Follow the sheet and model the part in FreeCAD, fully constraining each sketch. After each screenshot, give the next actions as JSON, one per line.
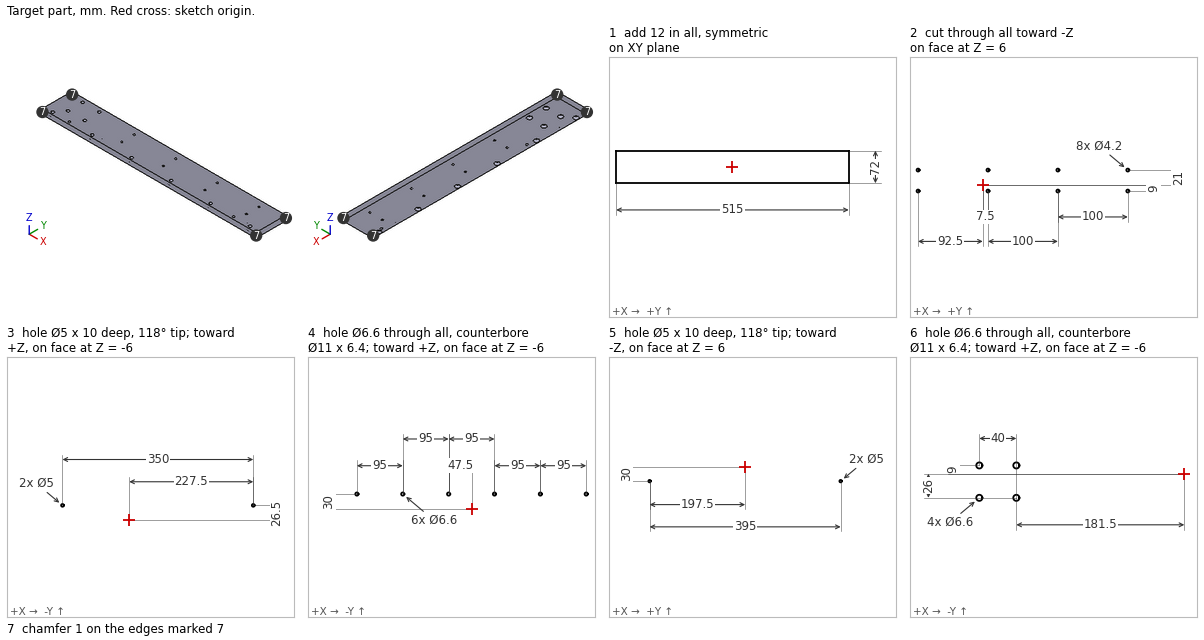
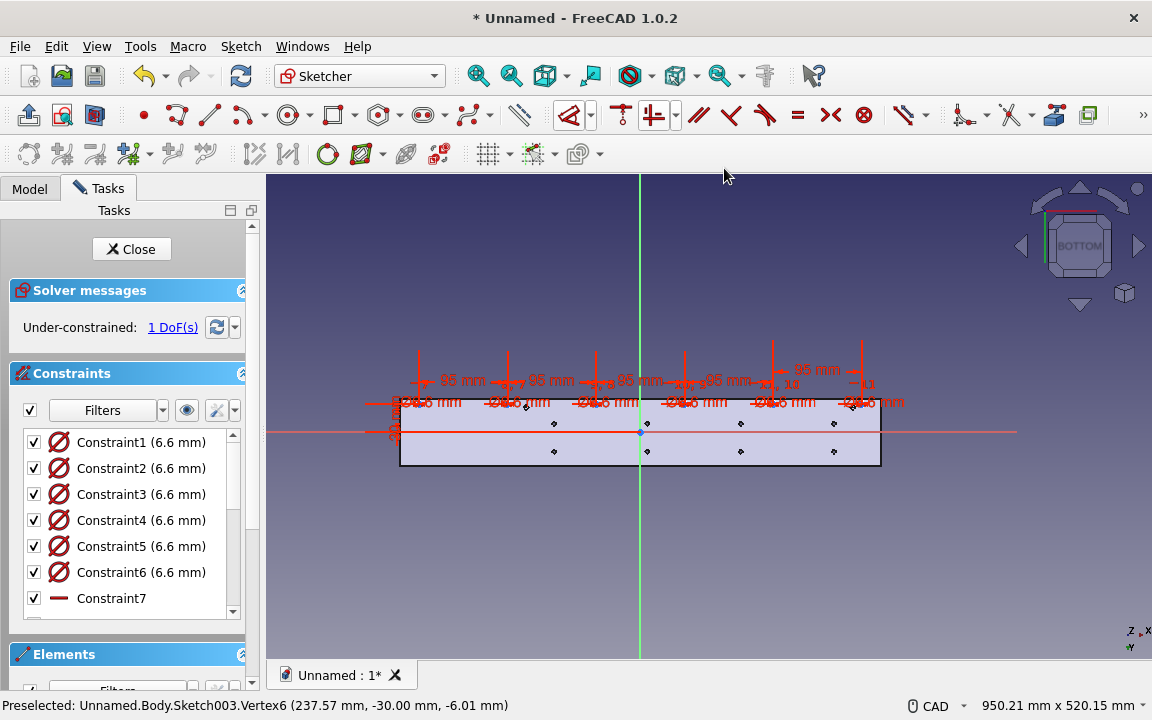
{"action": "left_click", "coordinate": [596, 404]}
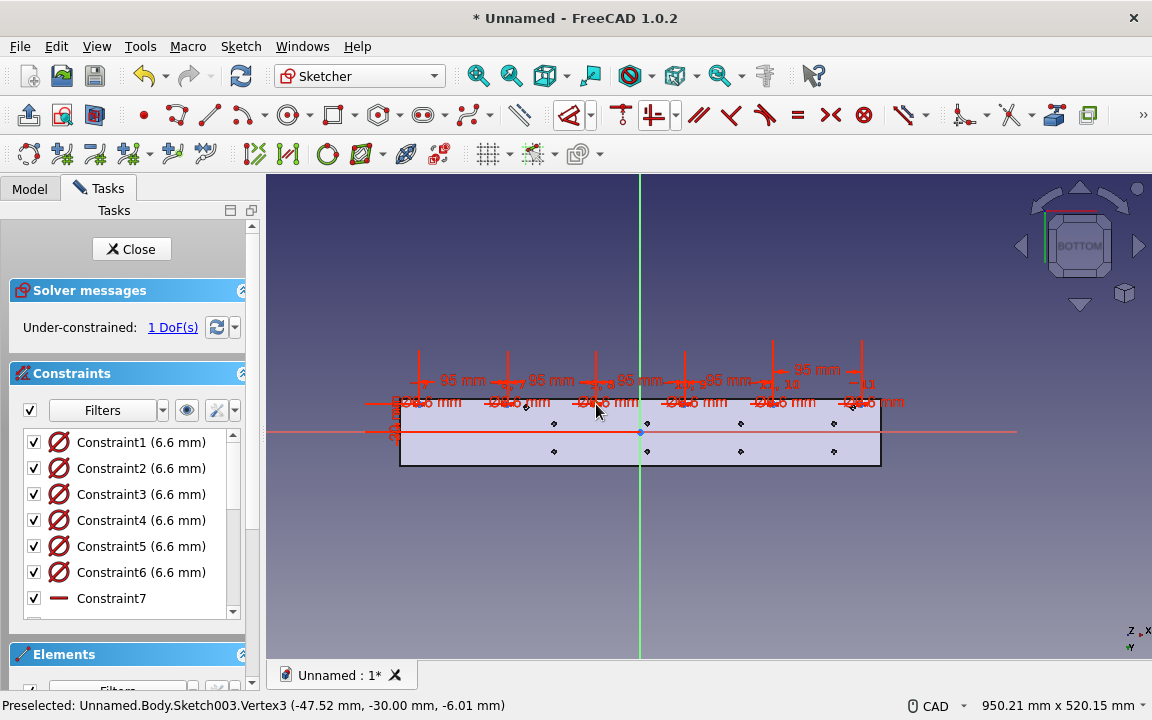
{"action": "left_click", "coordinate": [590, 116]}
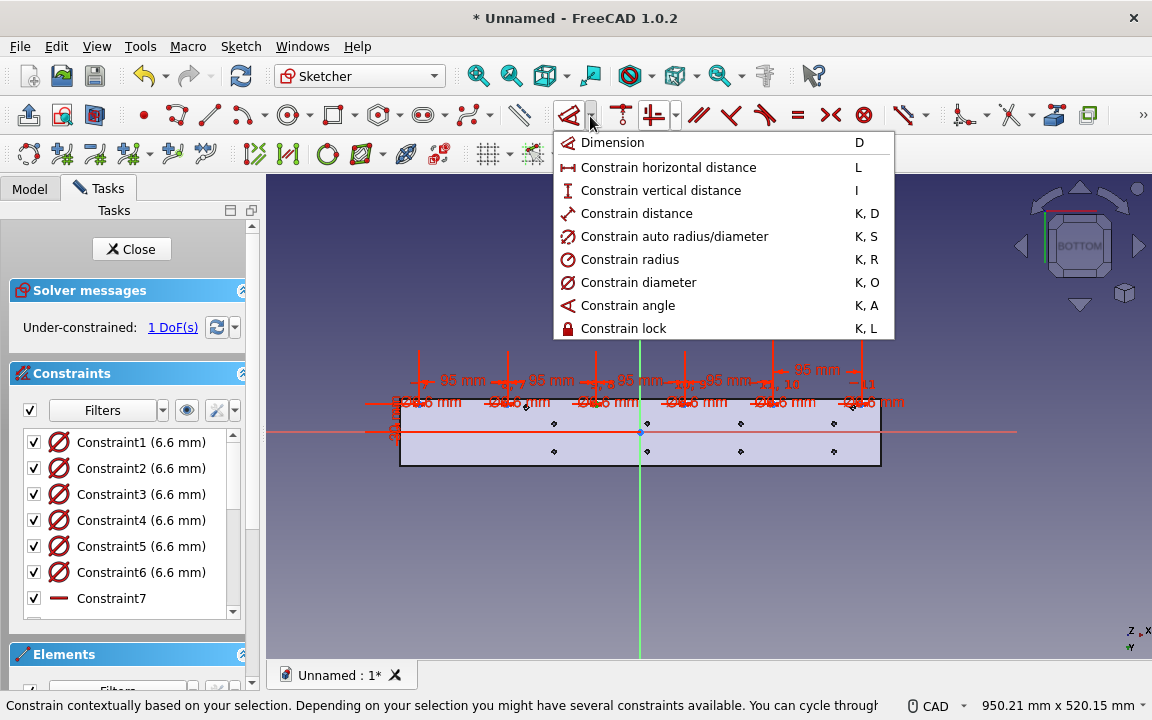
{"action": "left_click", "coordinate": [724, 168]}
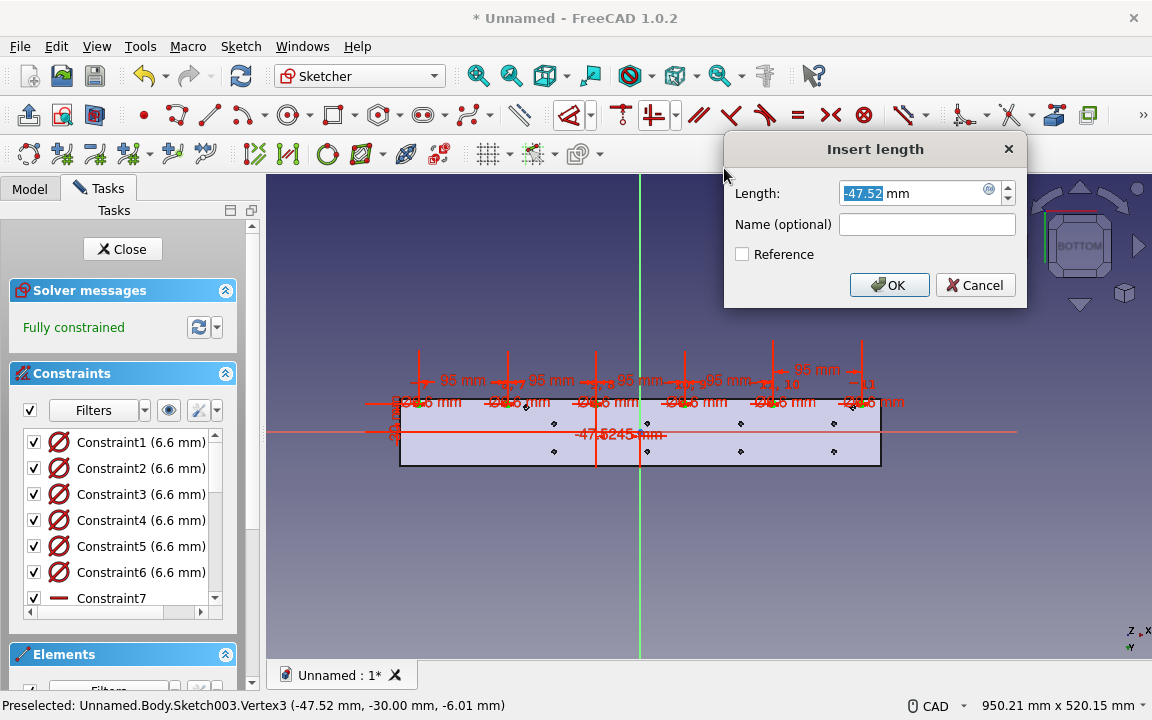
{"action": "type", "text": "-47.5"}
{"action": "key", "text": "Return"}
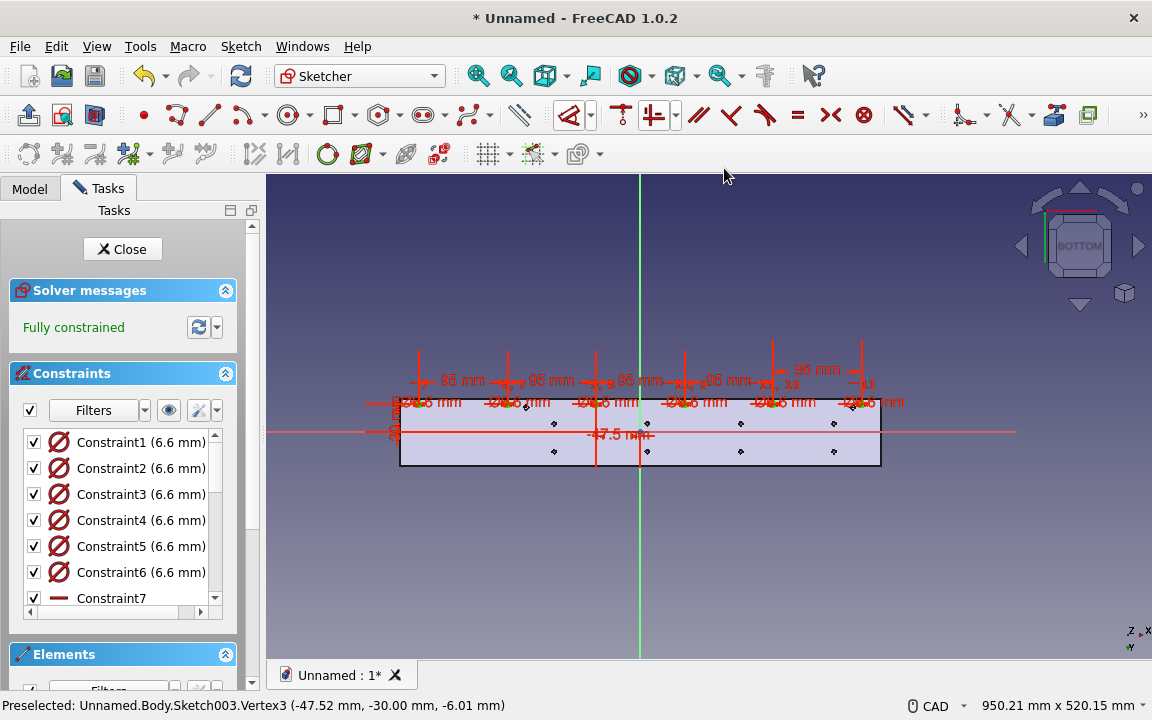
{"action": "left_click", "coordinate": [123, 249]}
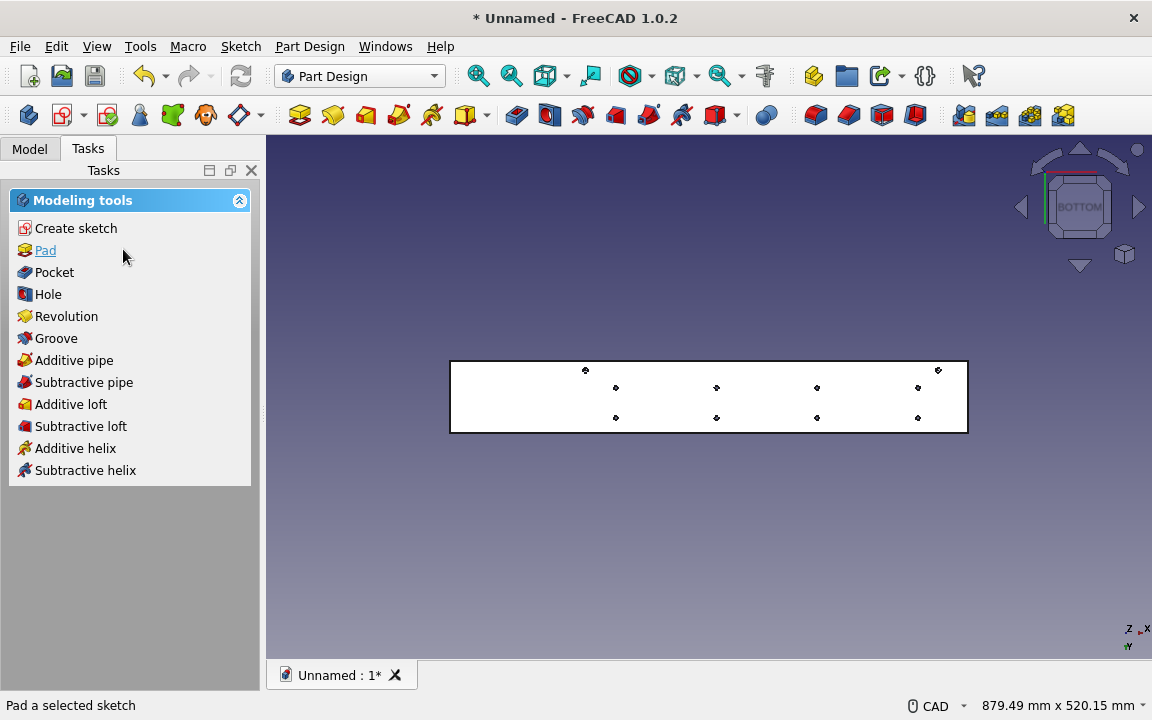
{"action": "left_click", "coordinate": [550, 116]}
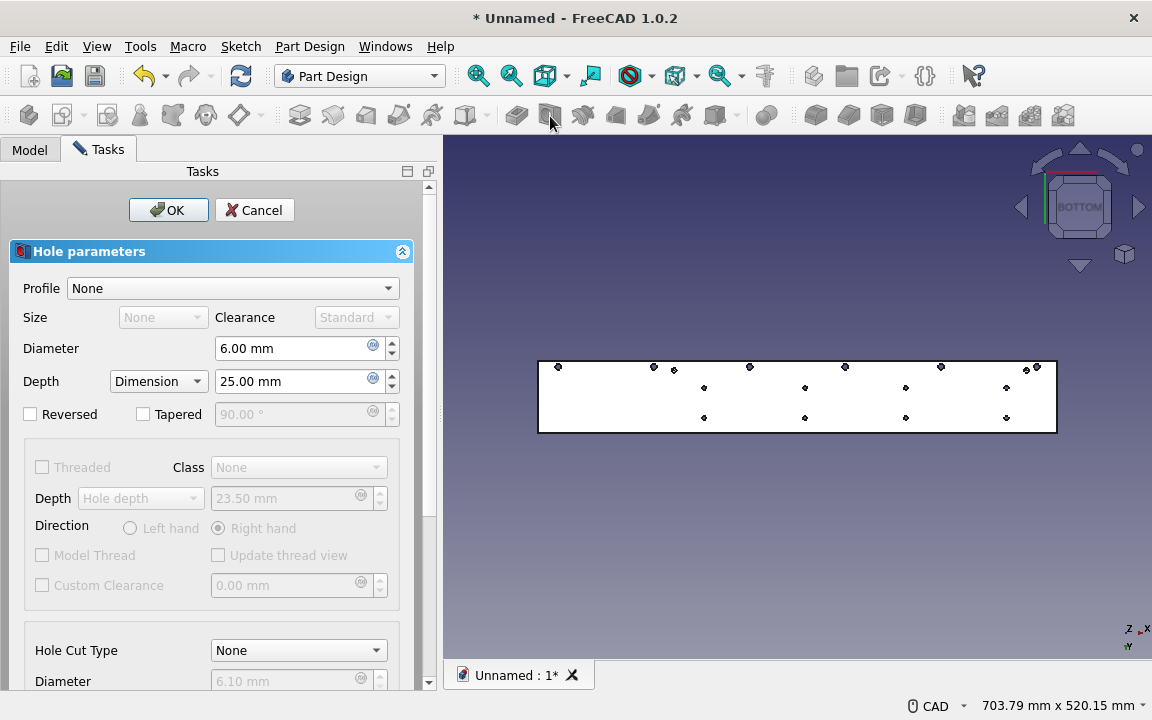
{"action": "triple_click", "coordinate": [300, 348]}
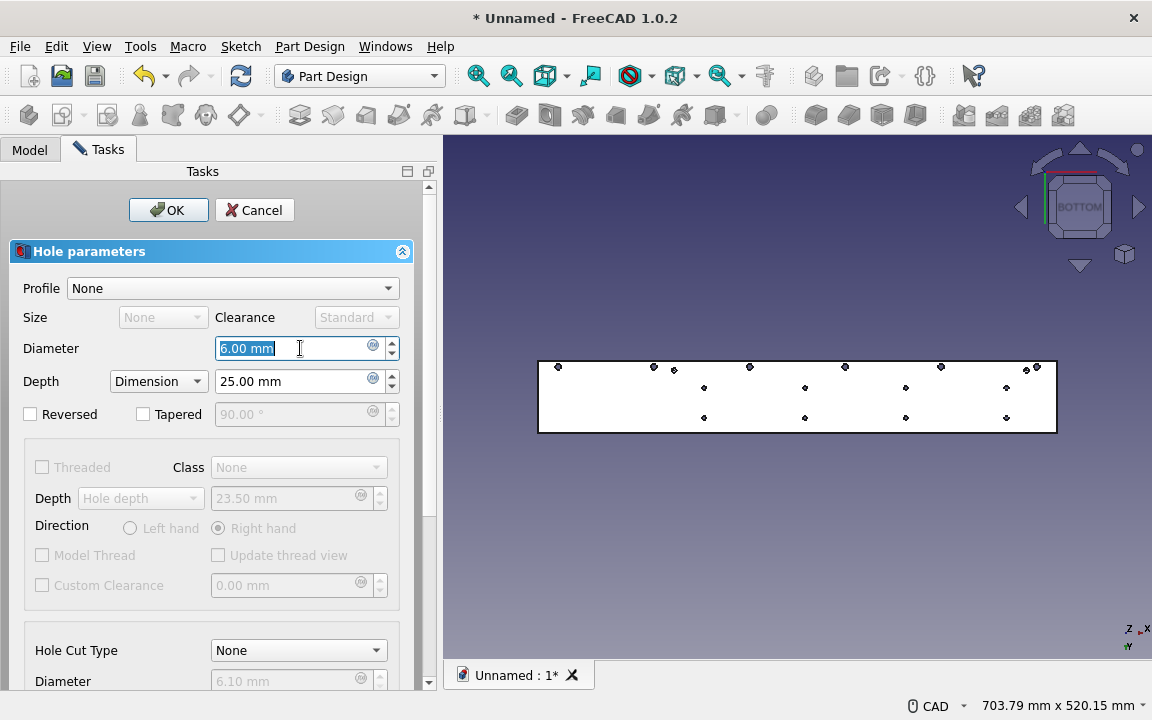
{"action": "type", "text": "6.6"}
{"action": "key", "text": "Tab"}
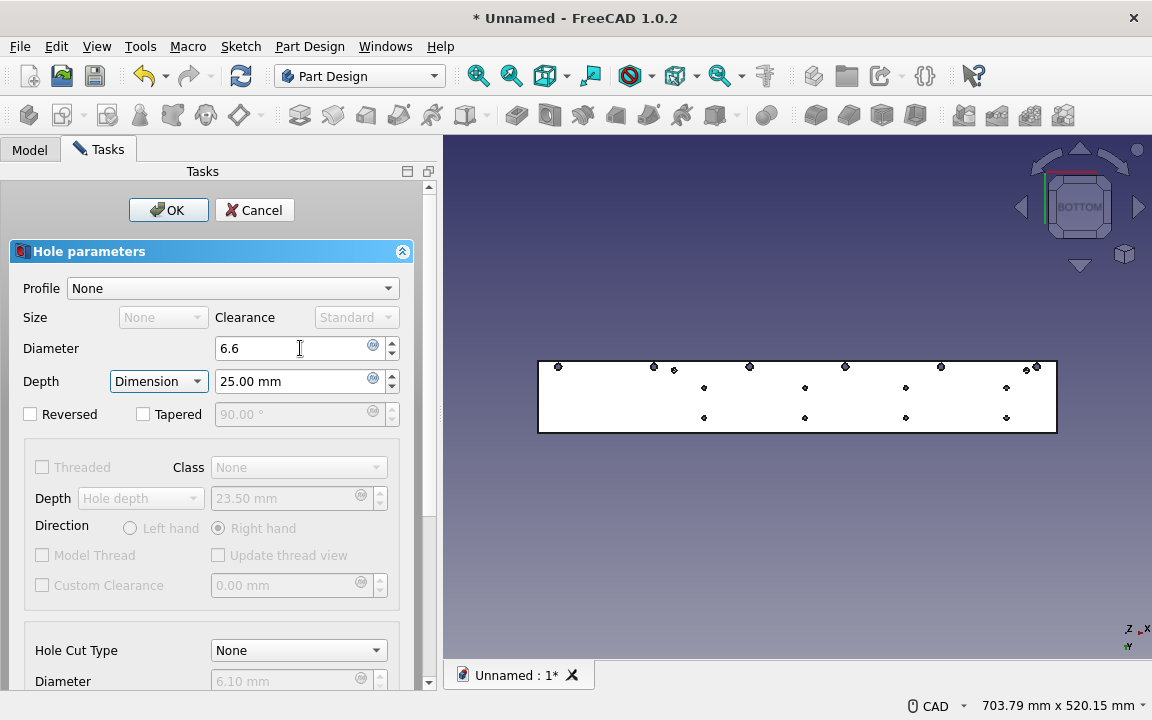
{"action": "left_click", "coordinate": [160, 382]}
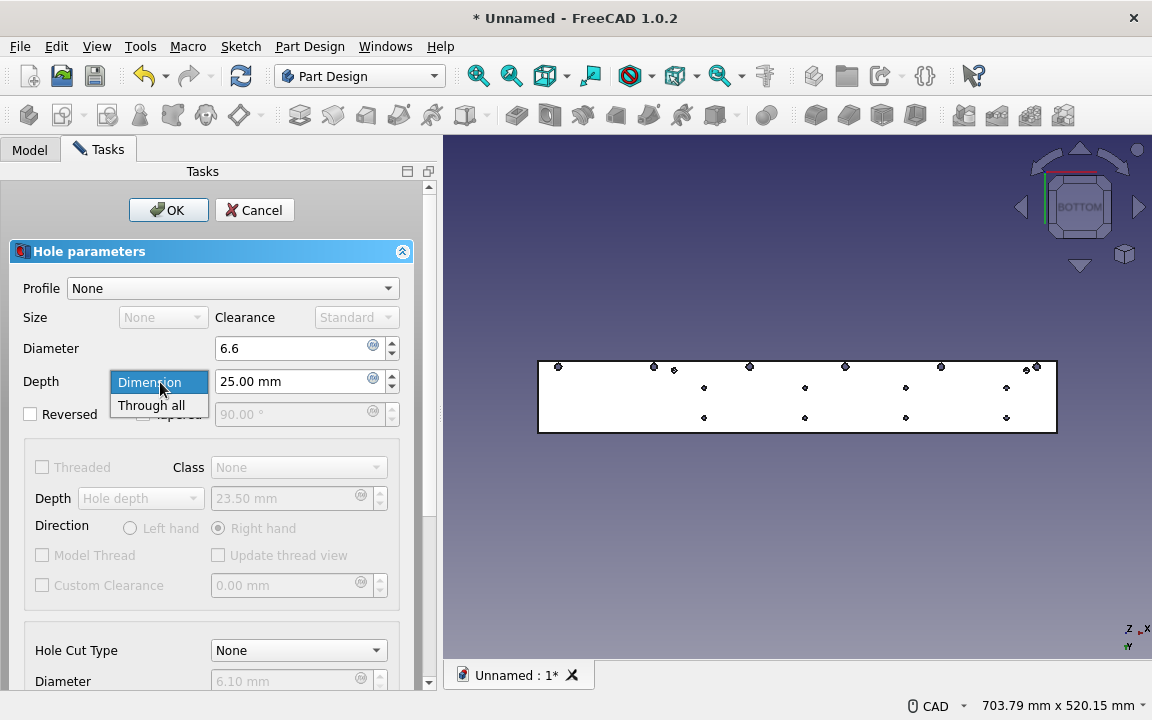
{"action": "left_click", "coordinate": [158, 406]}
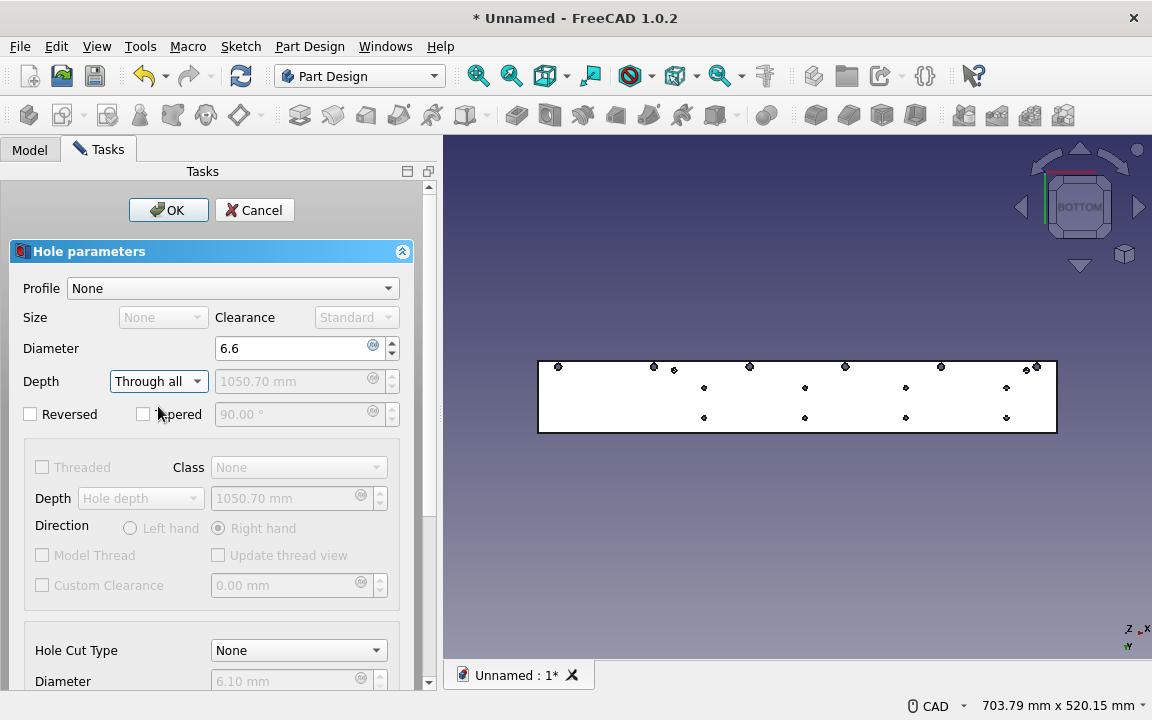
{"action": "left_click", "coordinate": [300, 650]}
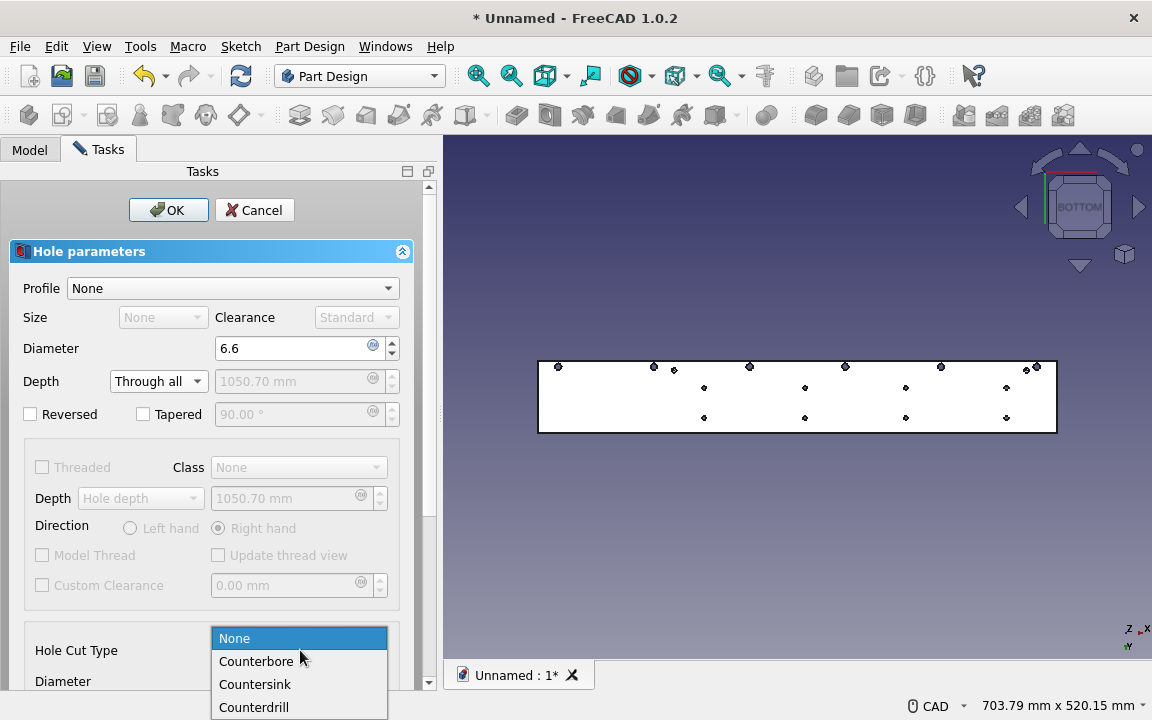
{"action": "left_click", "coordinate": [298, 662]}